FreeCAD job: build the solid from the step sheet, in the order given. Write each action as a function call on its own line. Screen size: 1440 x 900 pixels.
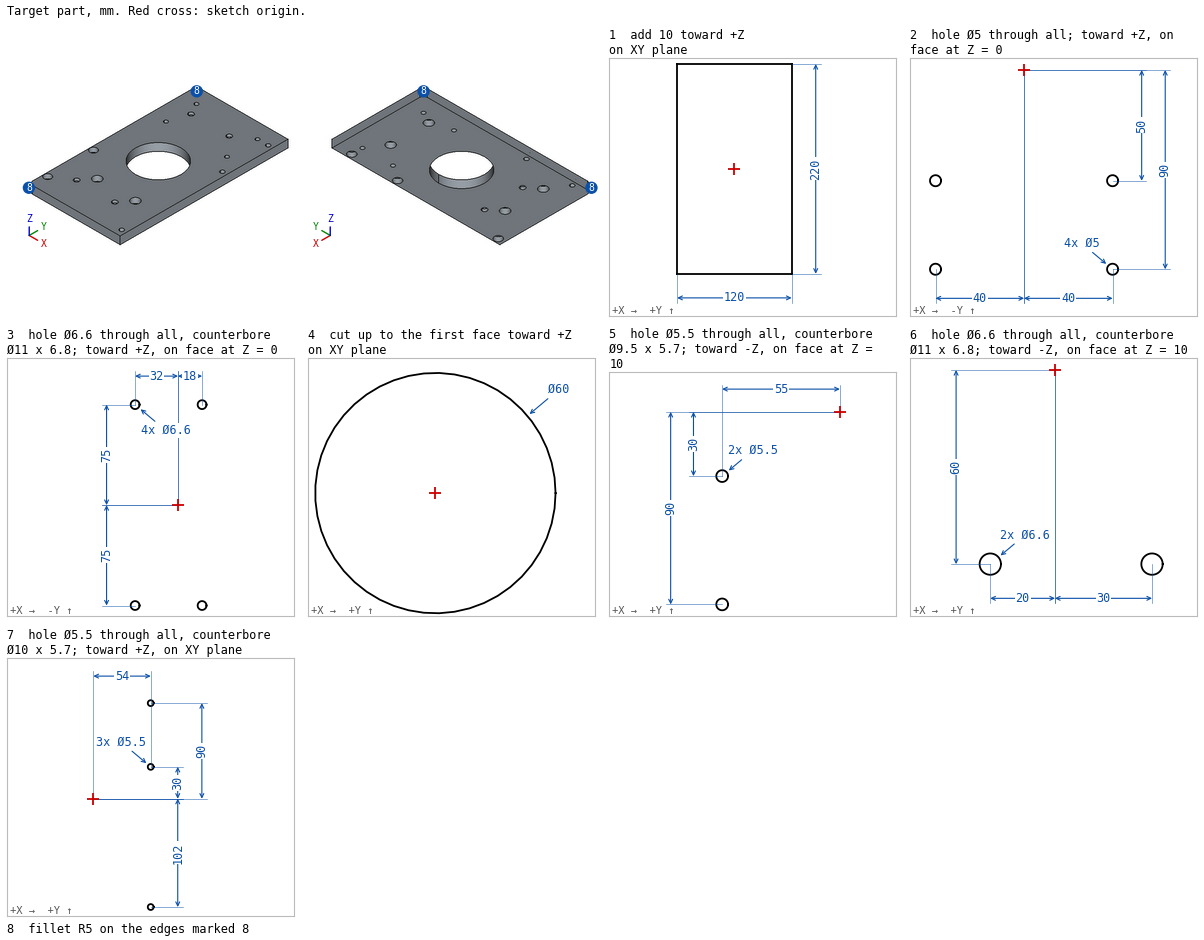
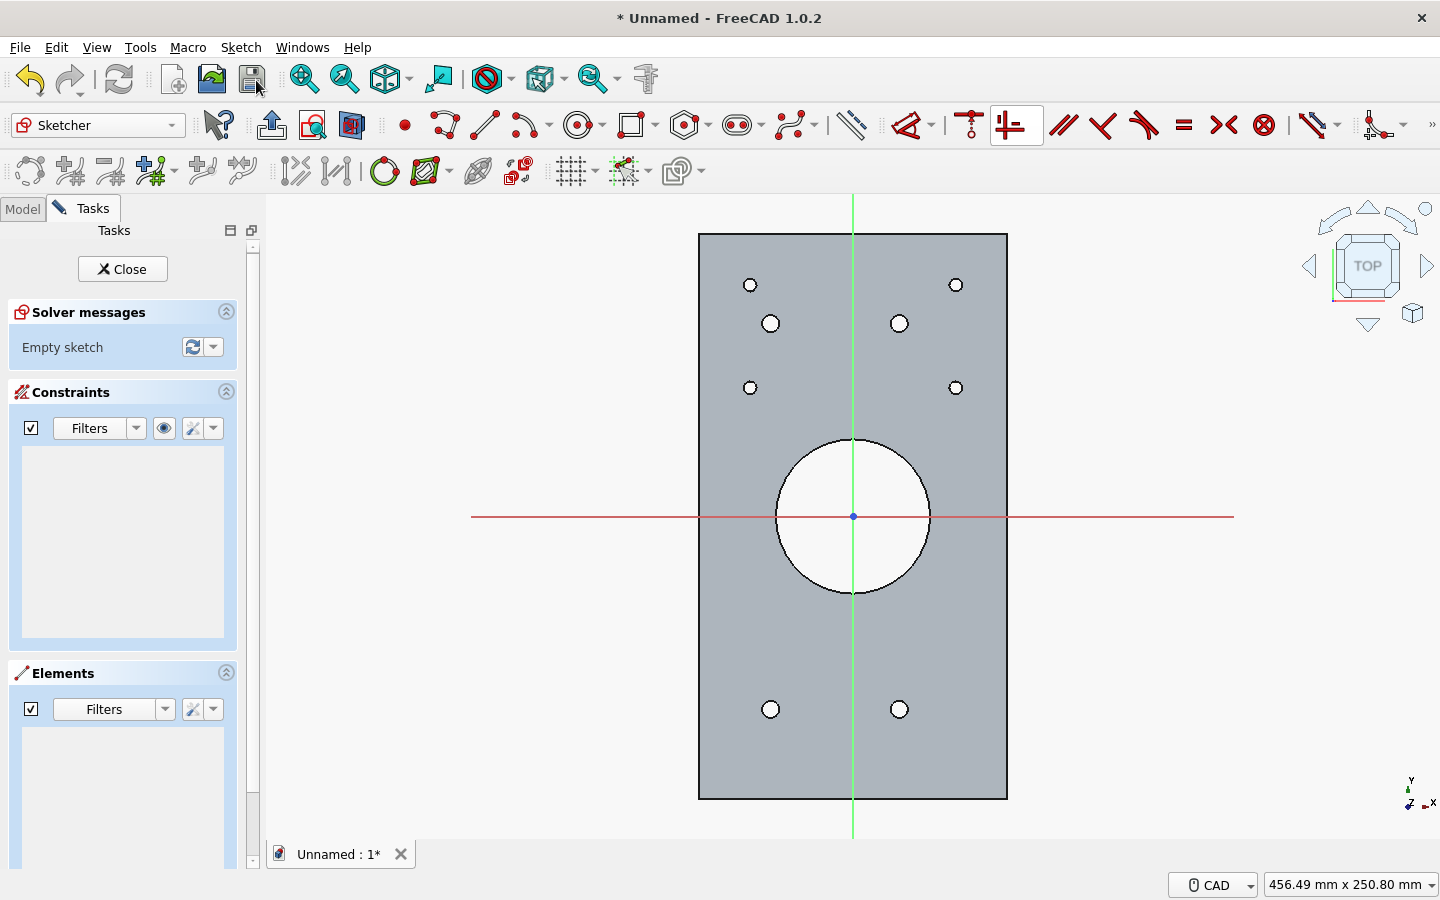
scroll(772, 781, up, 3)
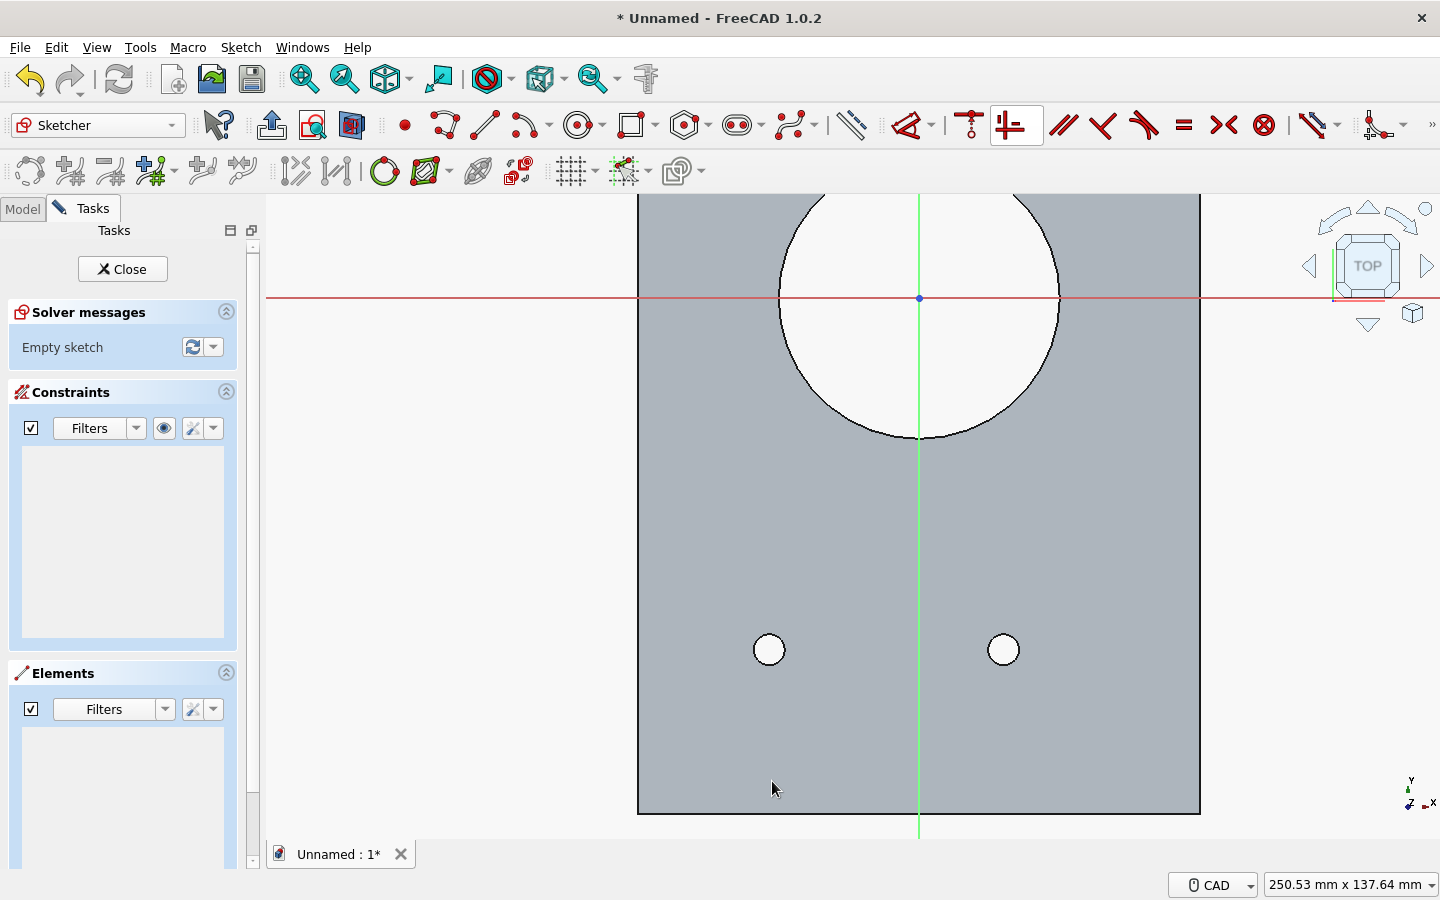
key(g)
key(c)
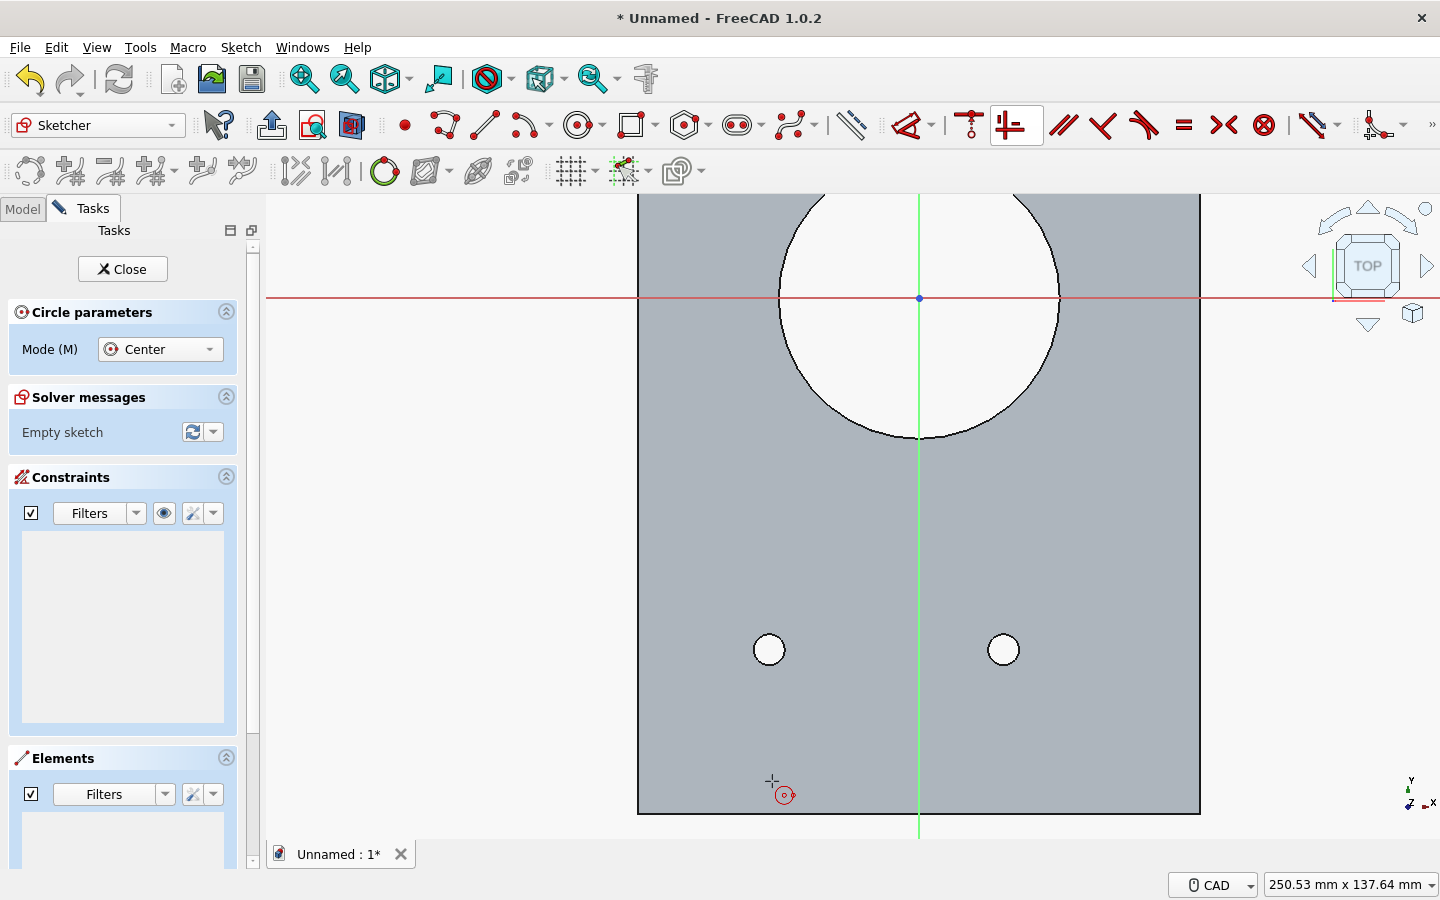
scroll(662, 439, up, 3)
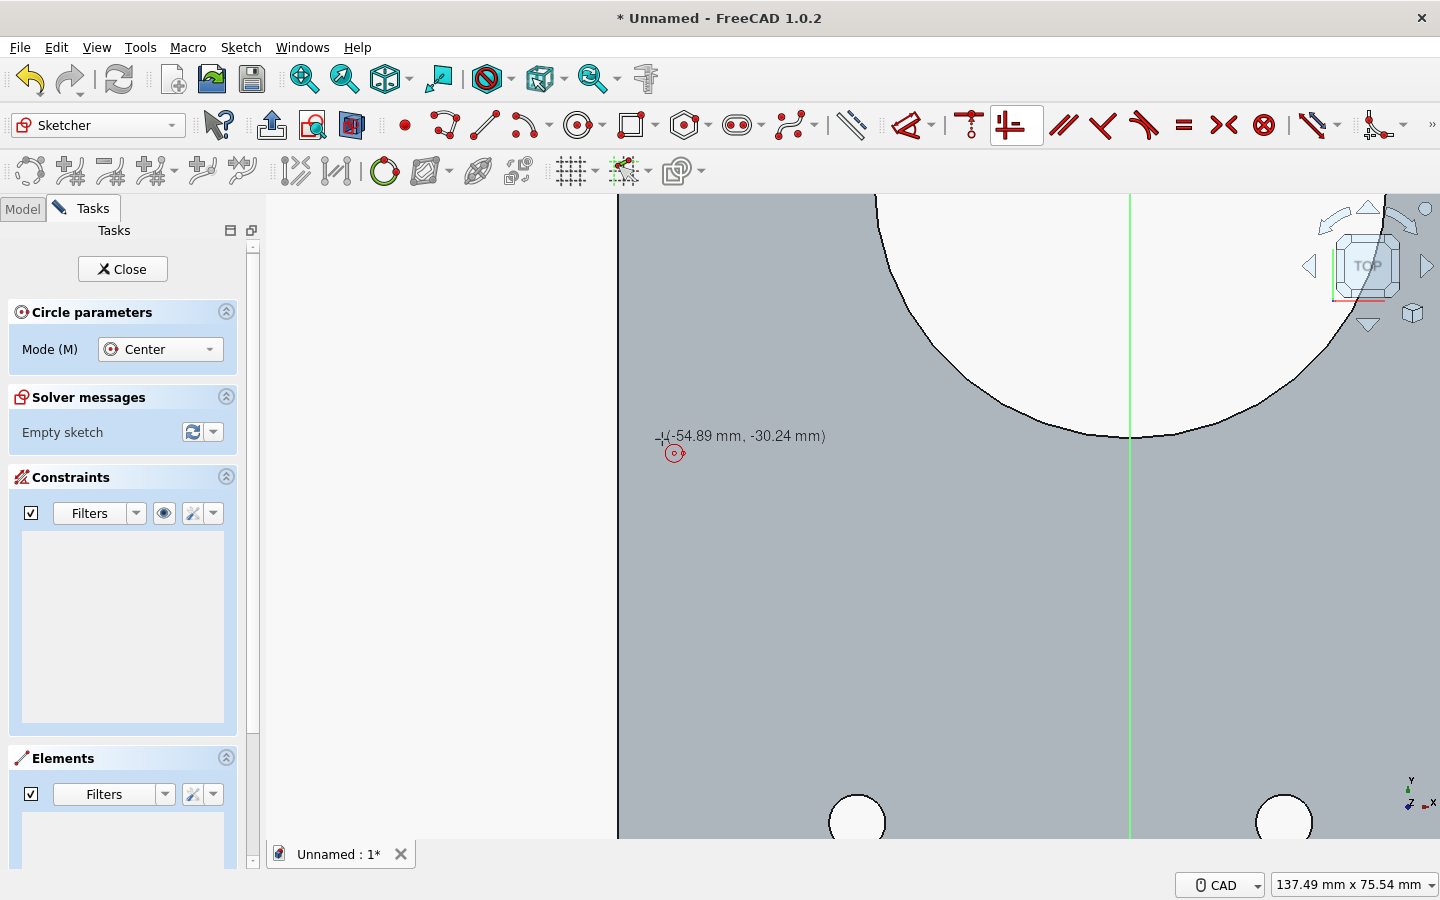
click(661, 438)
move(677, 422)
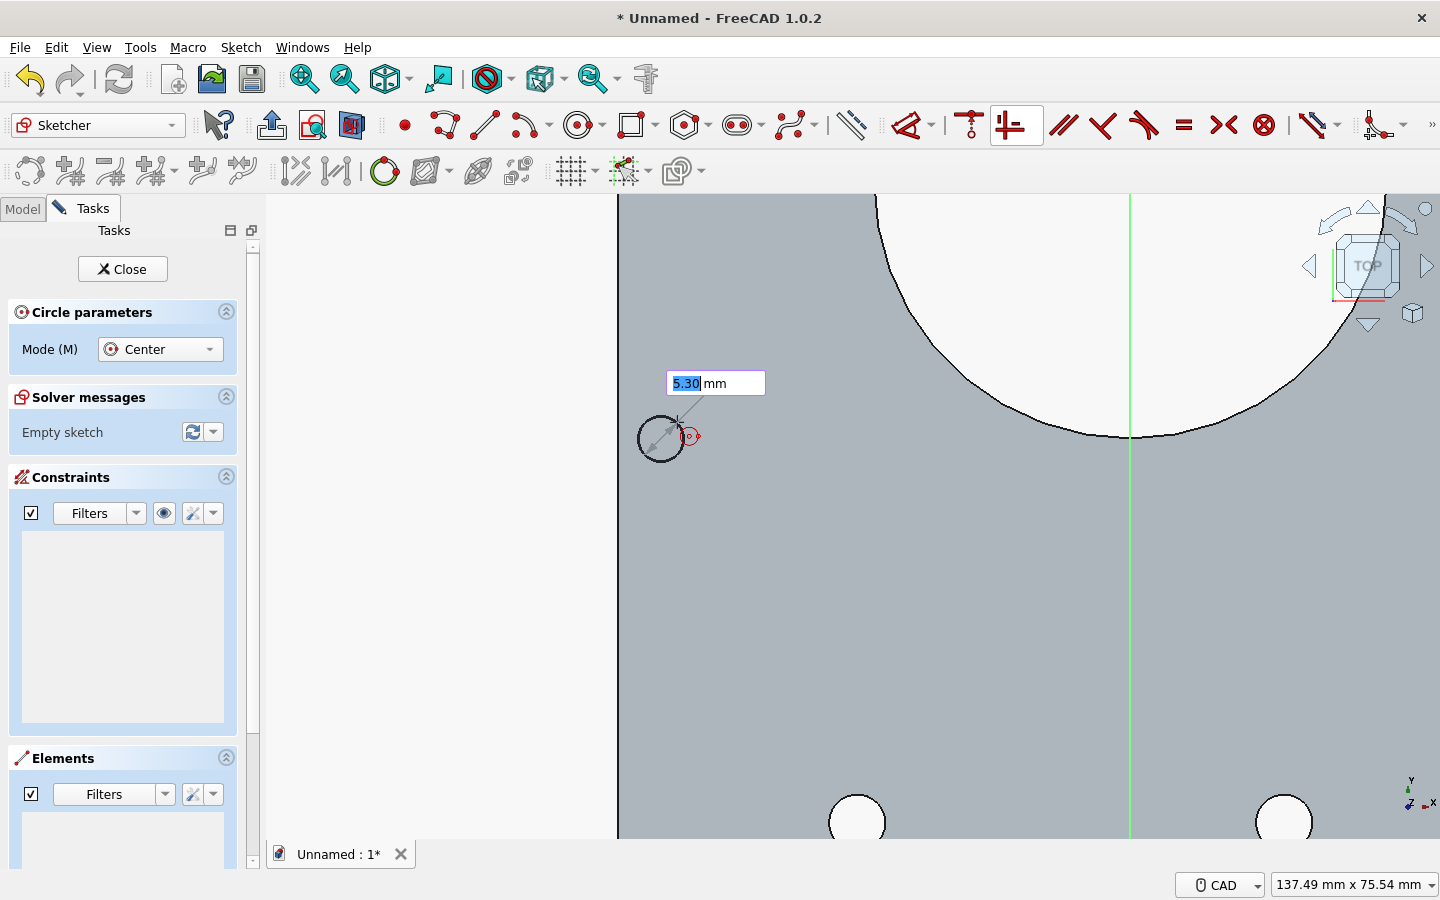
text(5.5)
key(Return)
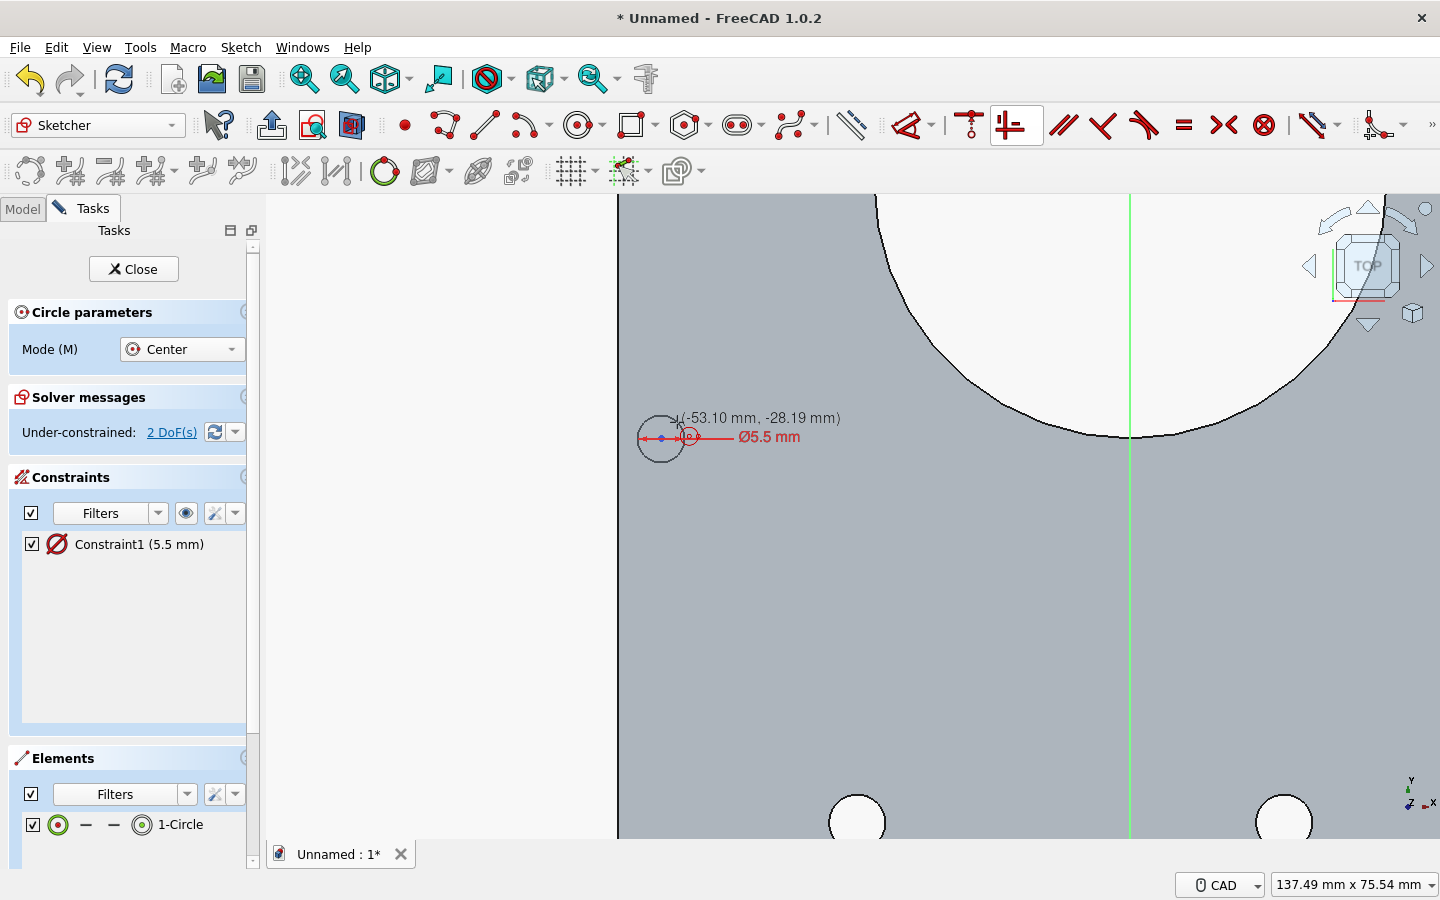
scroll(664, 441, down, 3)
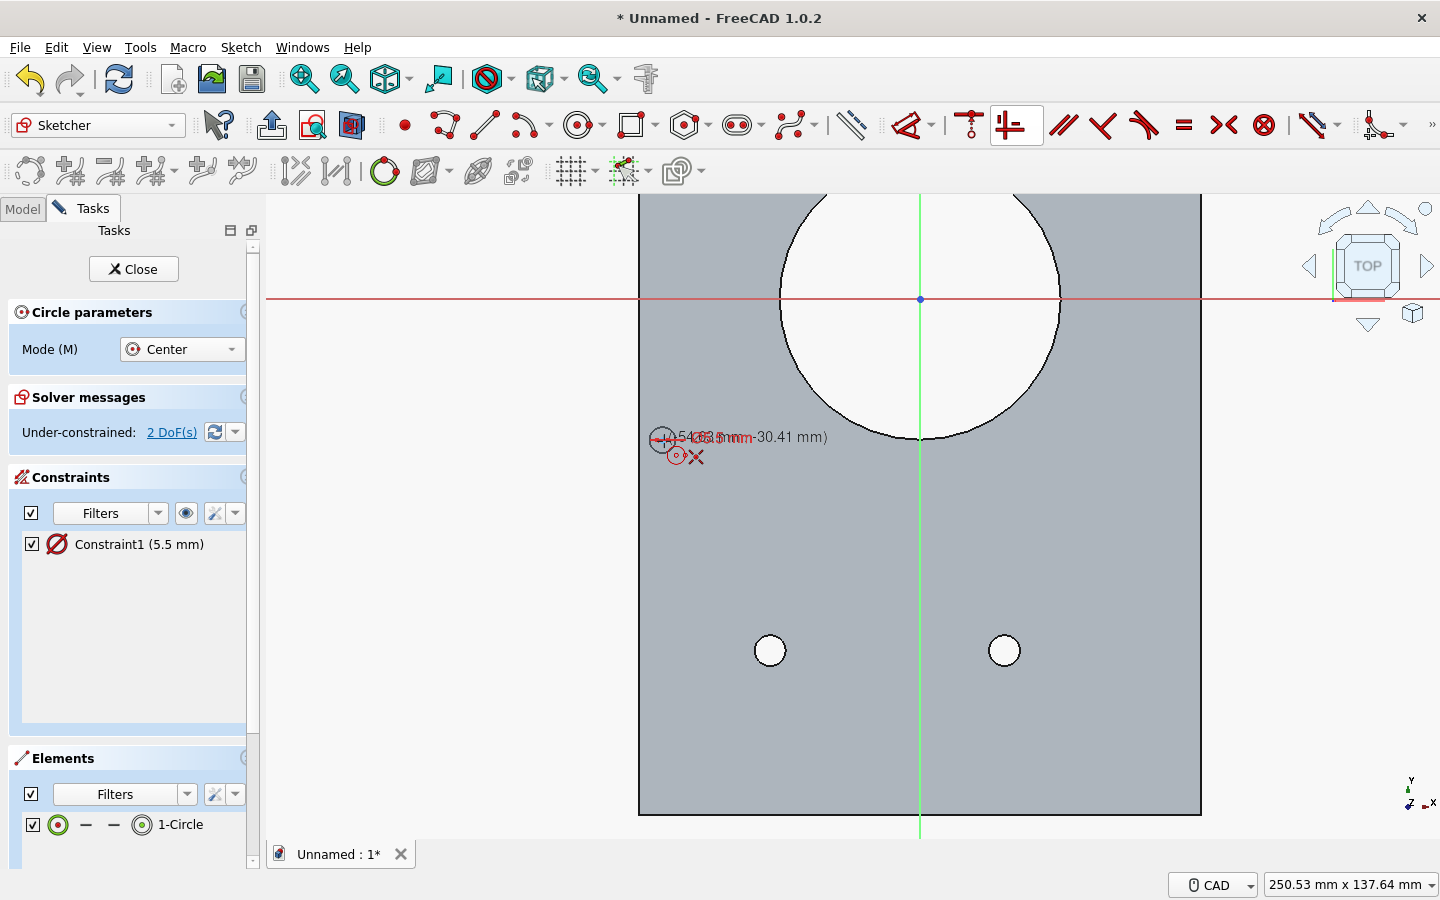
scroll(662, 721, up, 3)